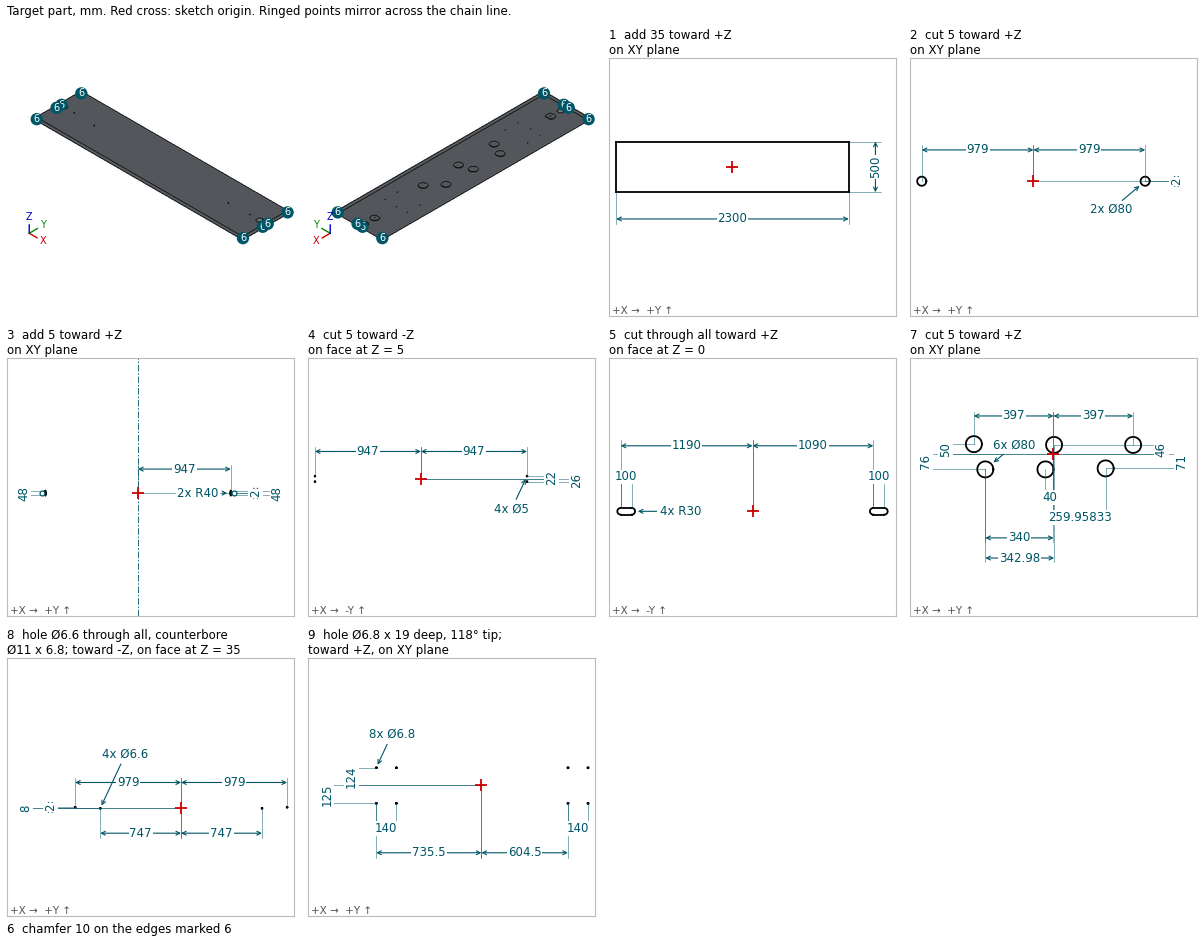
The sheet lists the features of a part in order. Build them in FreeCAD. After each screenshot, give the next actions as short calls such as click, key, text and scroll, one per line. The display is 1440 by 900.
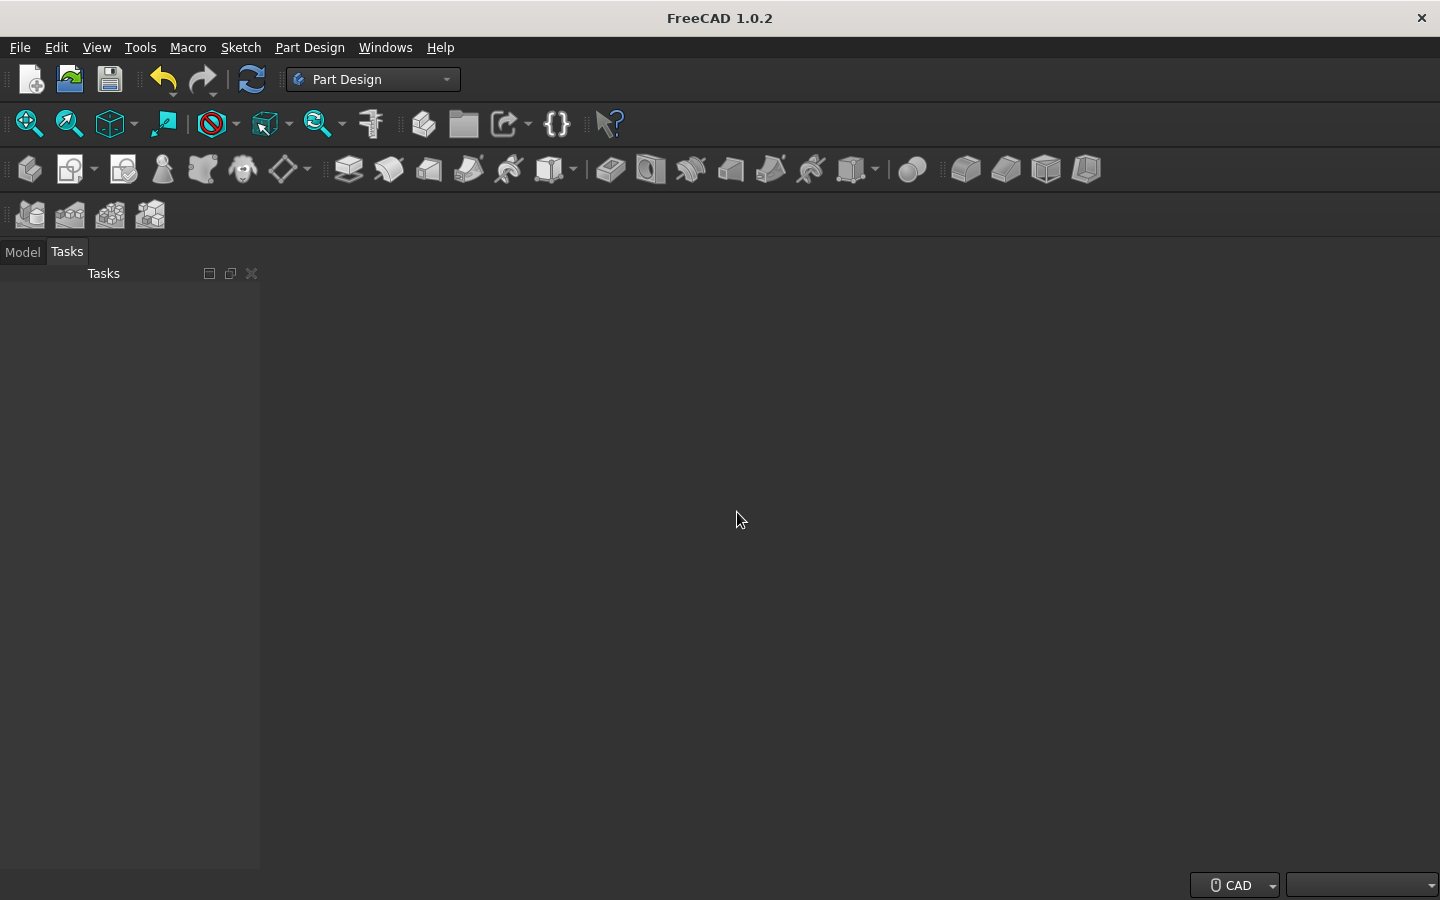
click(30, 80)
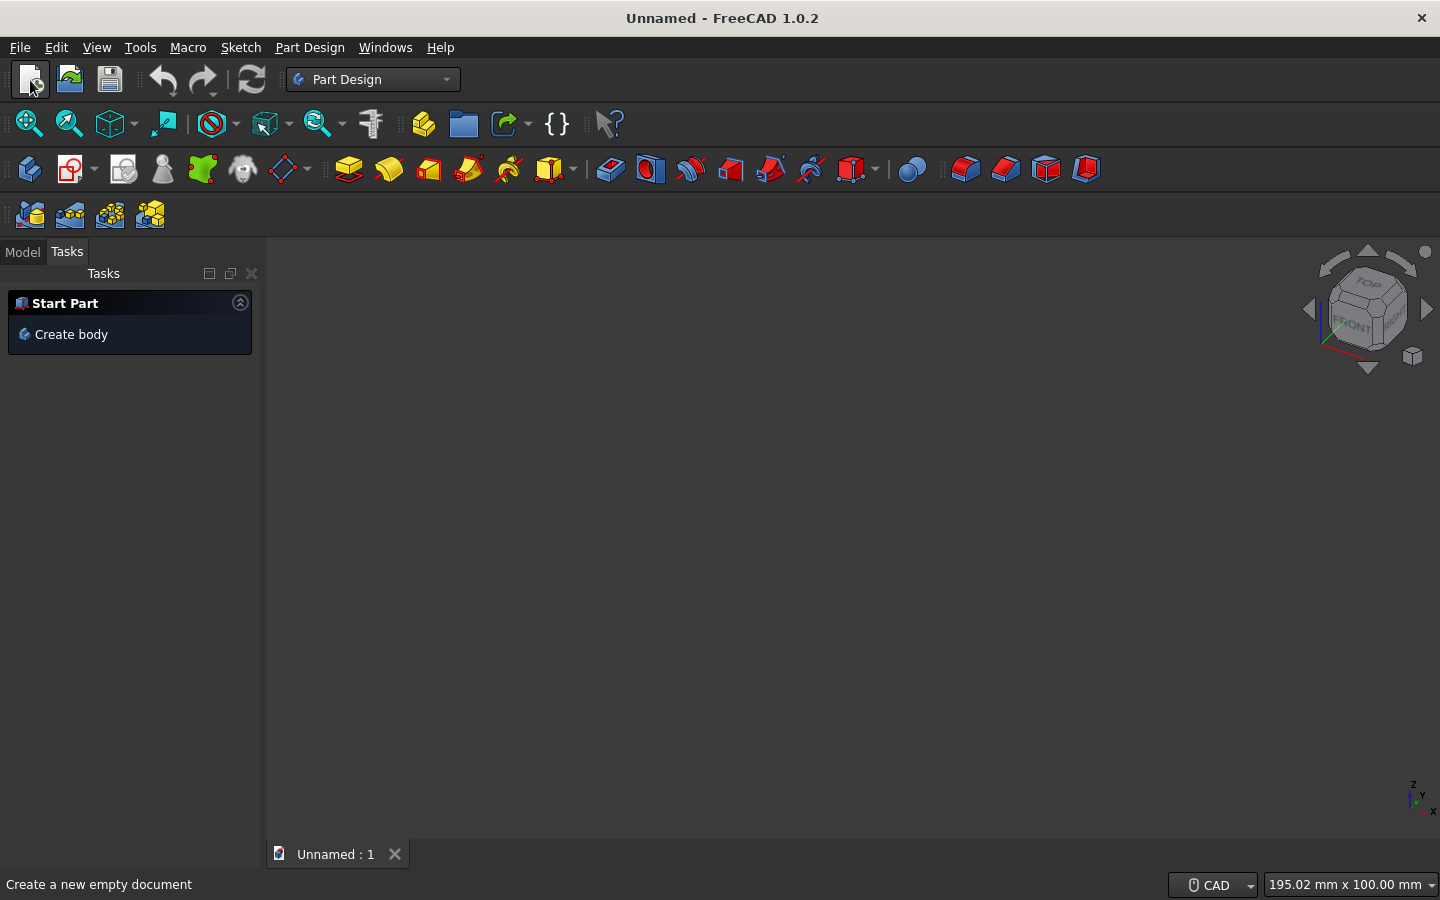
click(70, 170)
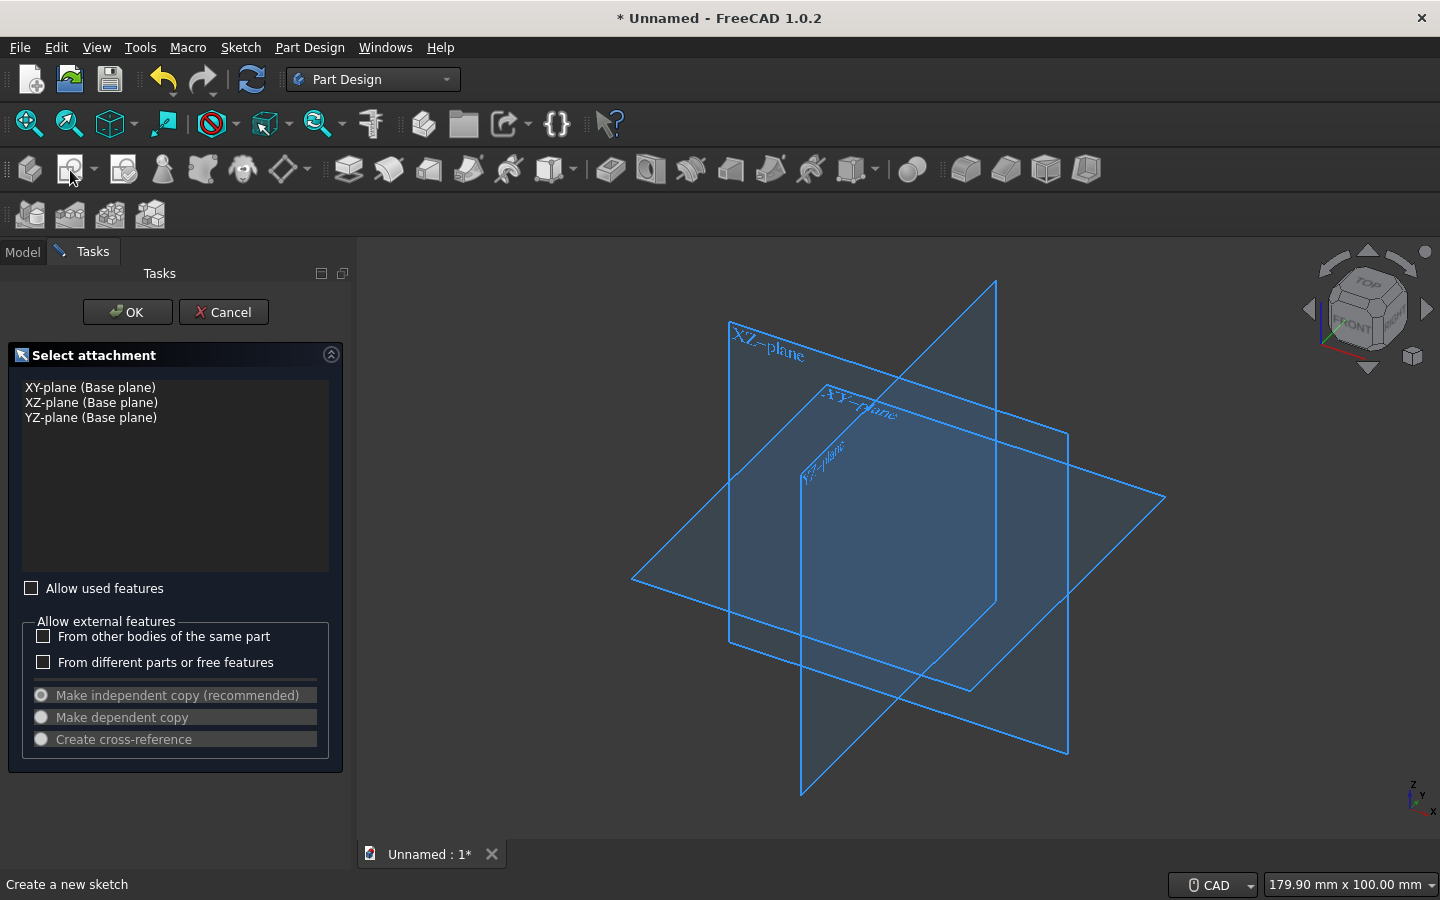
click(82, 388)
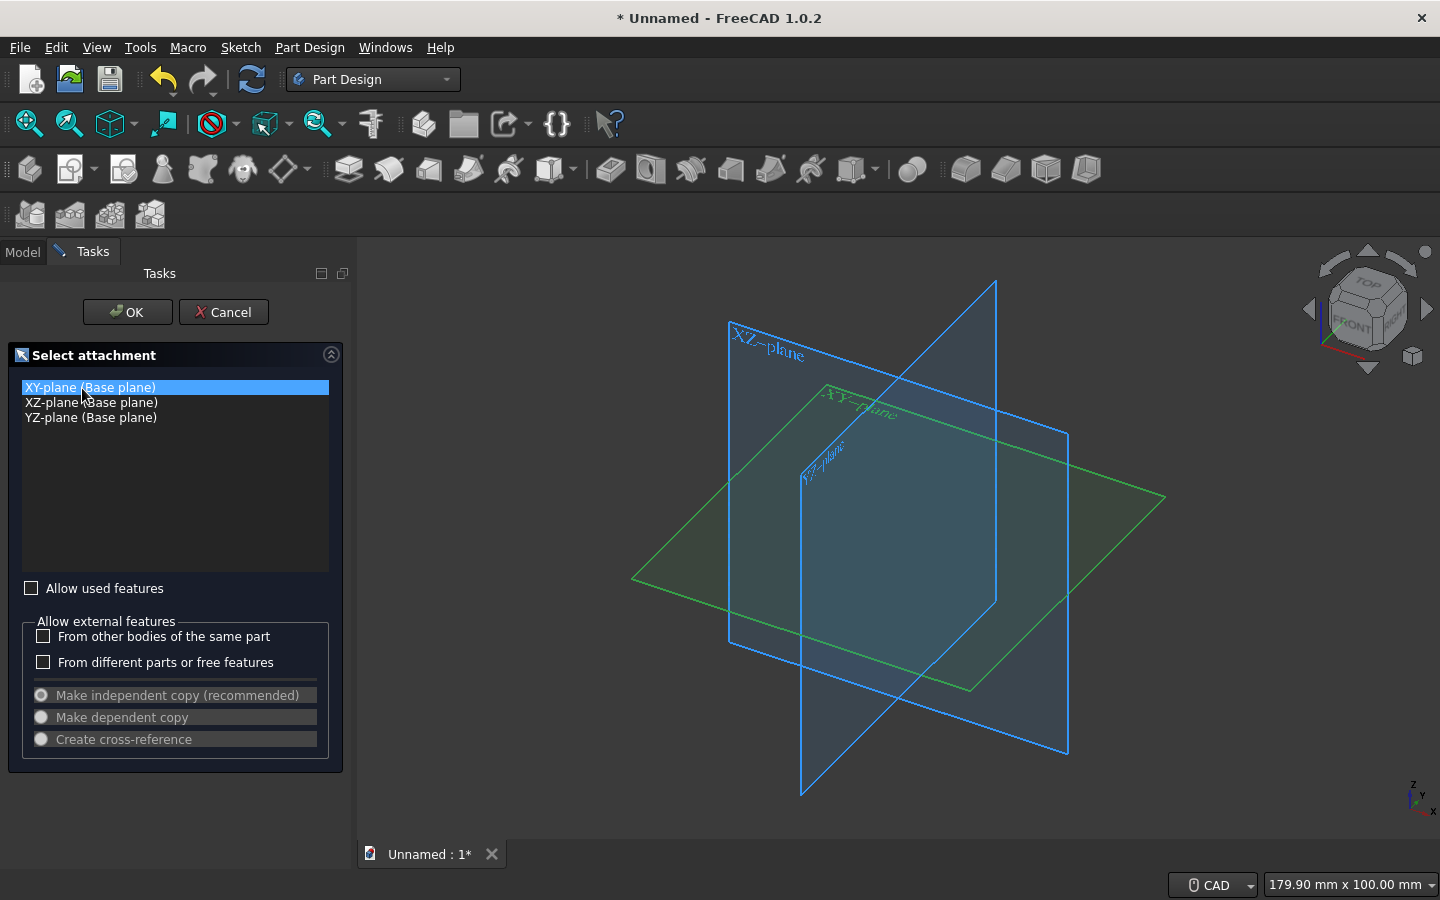
click(128, 312)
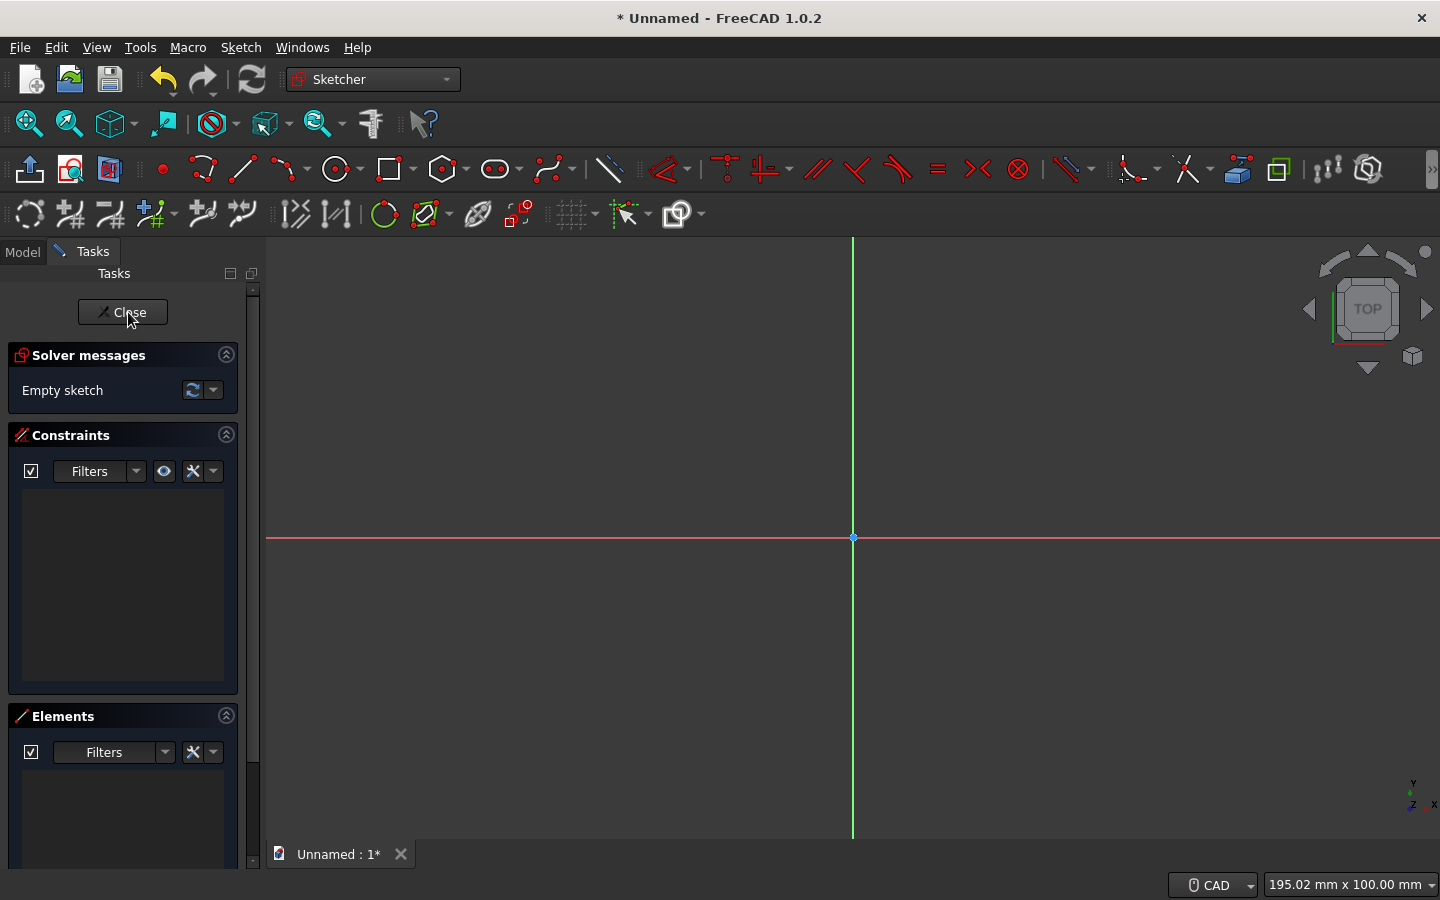
scroll(781, 538, down, 15)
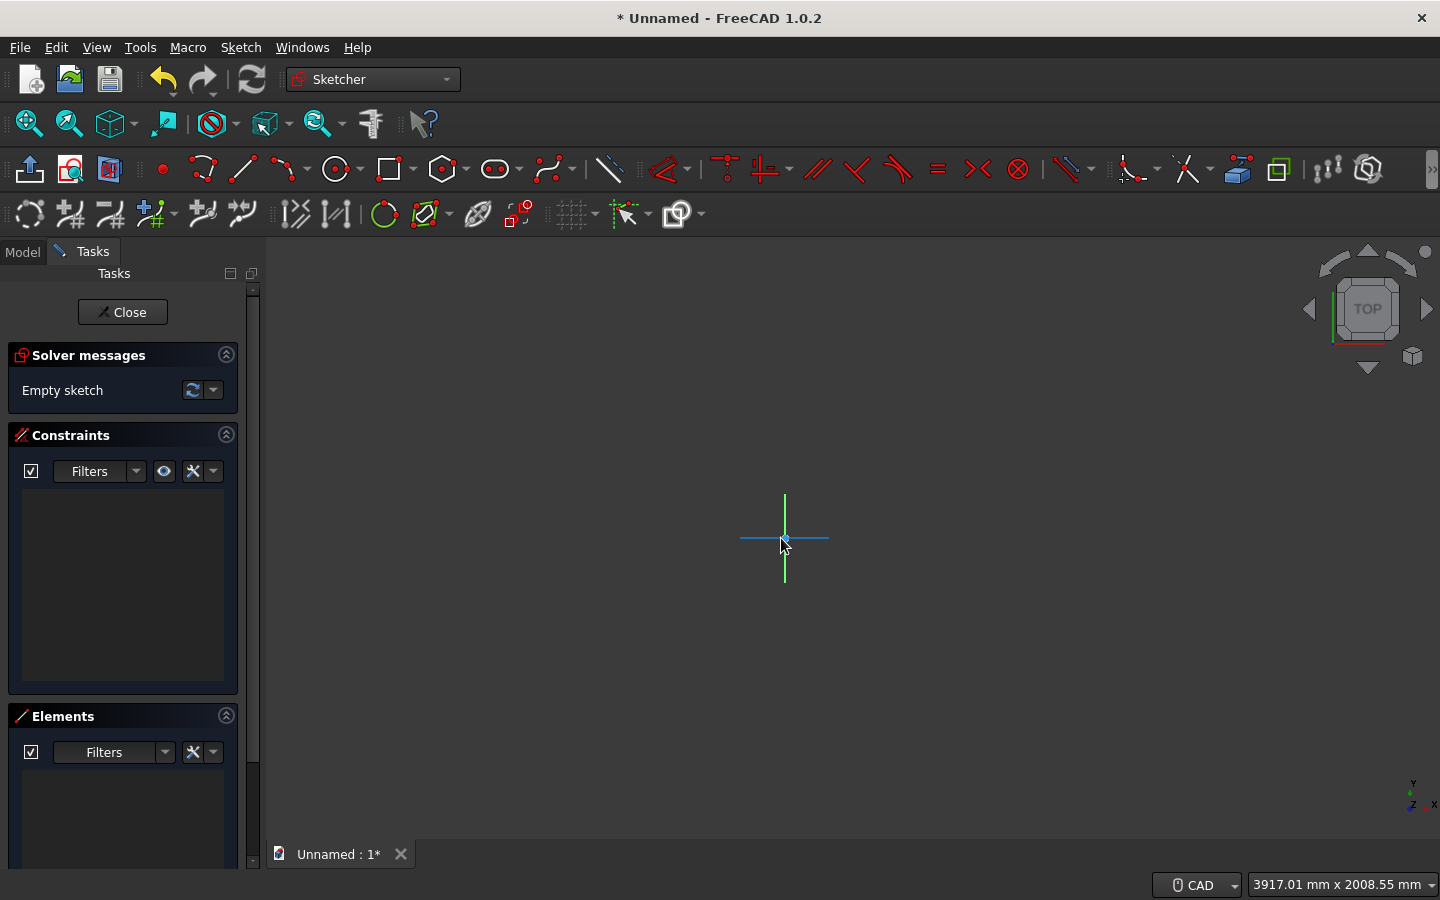
click(416, 170)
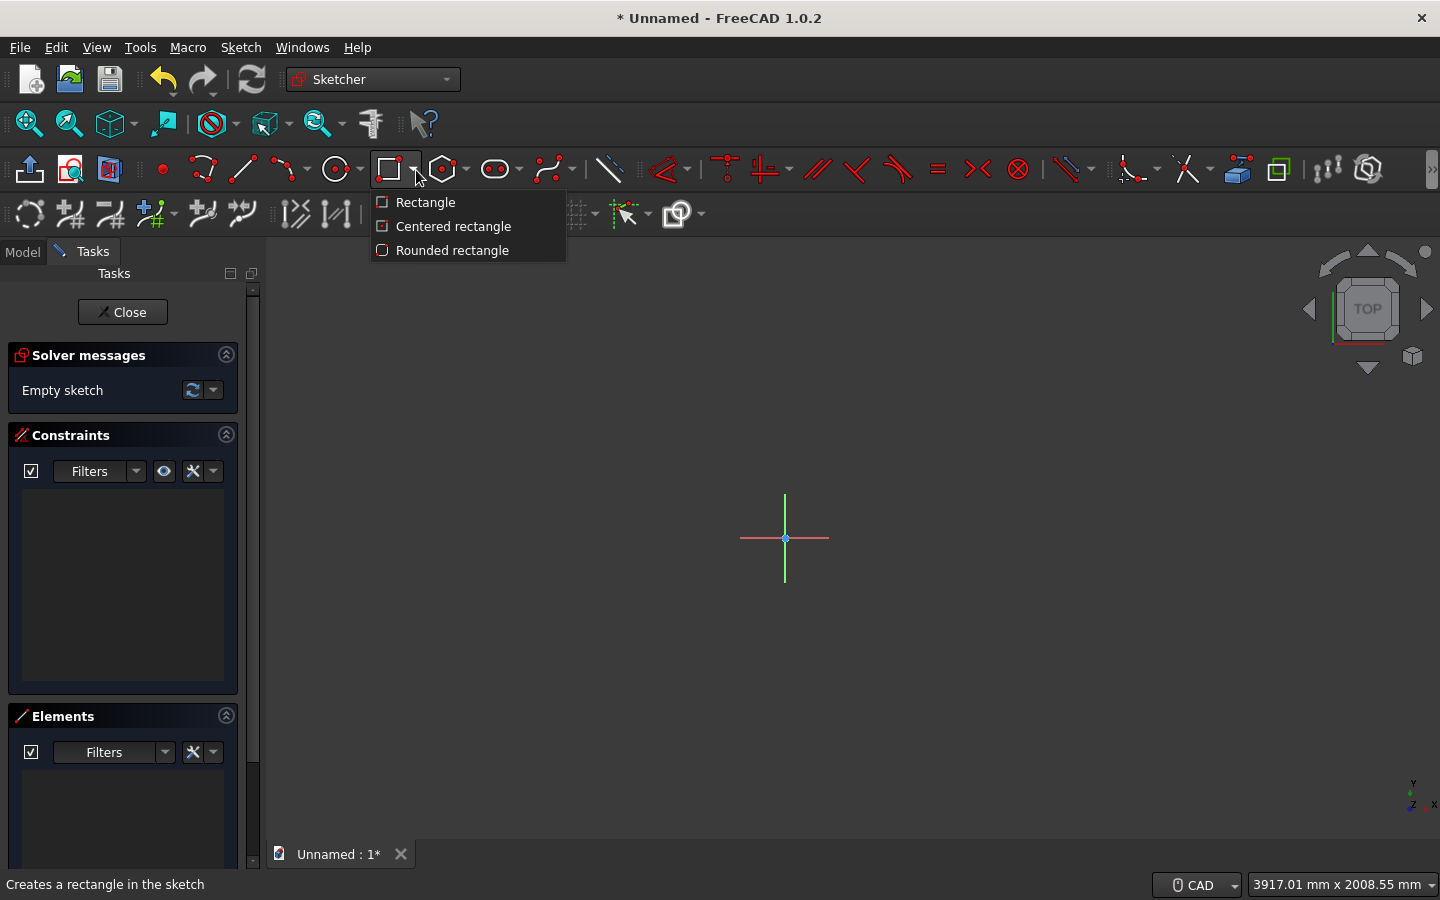
click(468, 226)